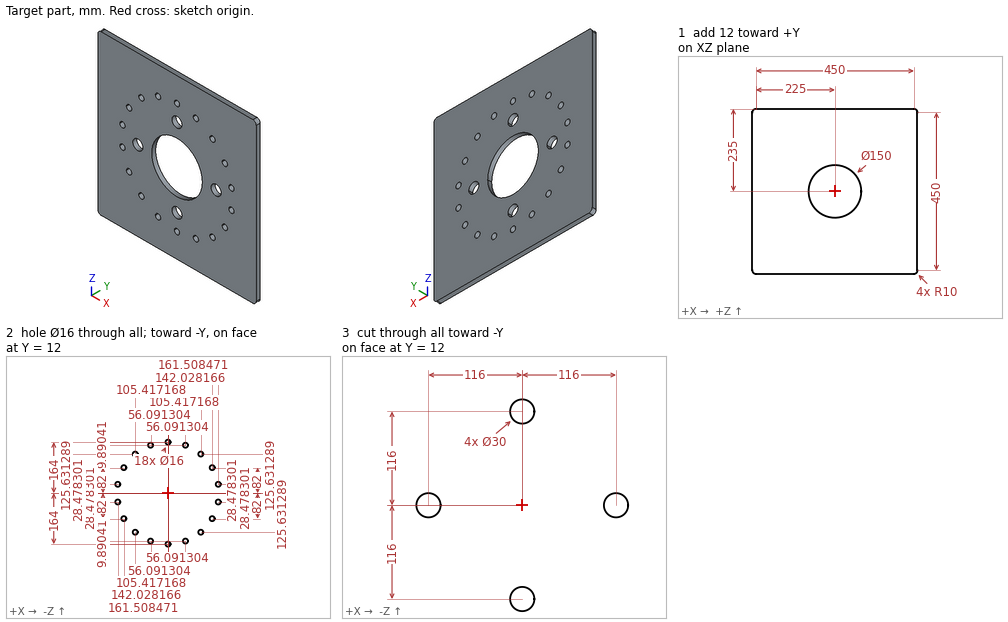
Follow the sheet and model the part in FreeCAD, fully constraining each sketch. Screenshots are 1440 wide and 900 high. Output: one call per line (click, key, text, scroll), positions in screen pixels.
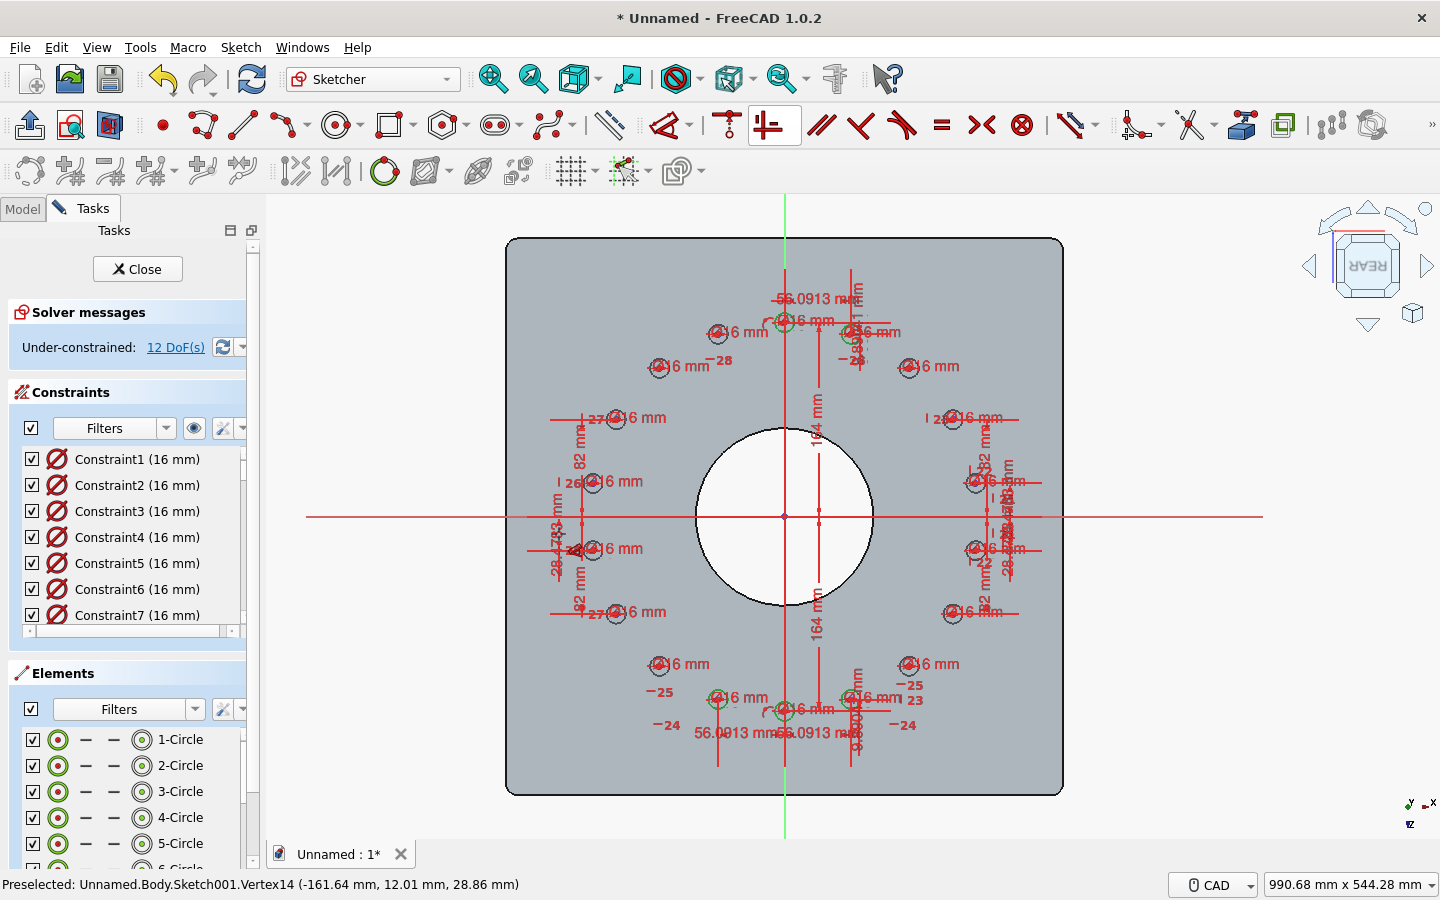
click(593, 483)
click(559, 500)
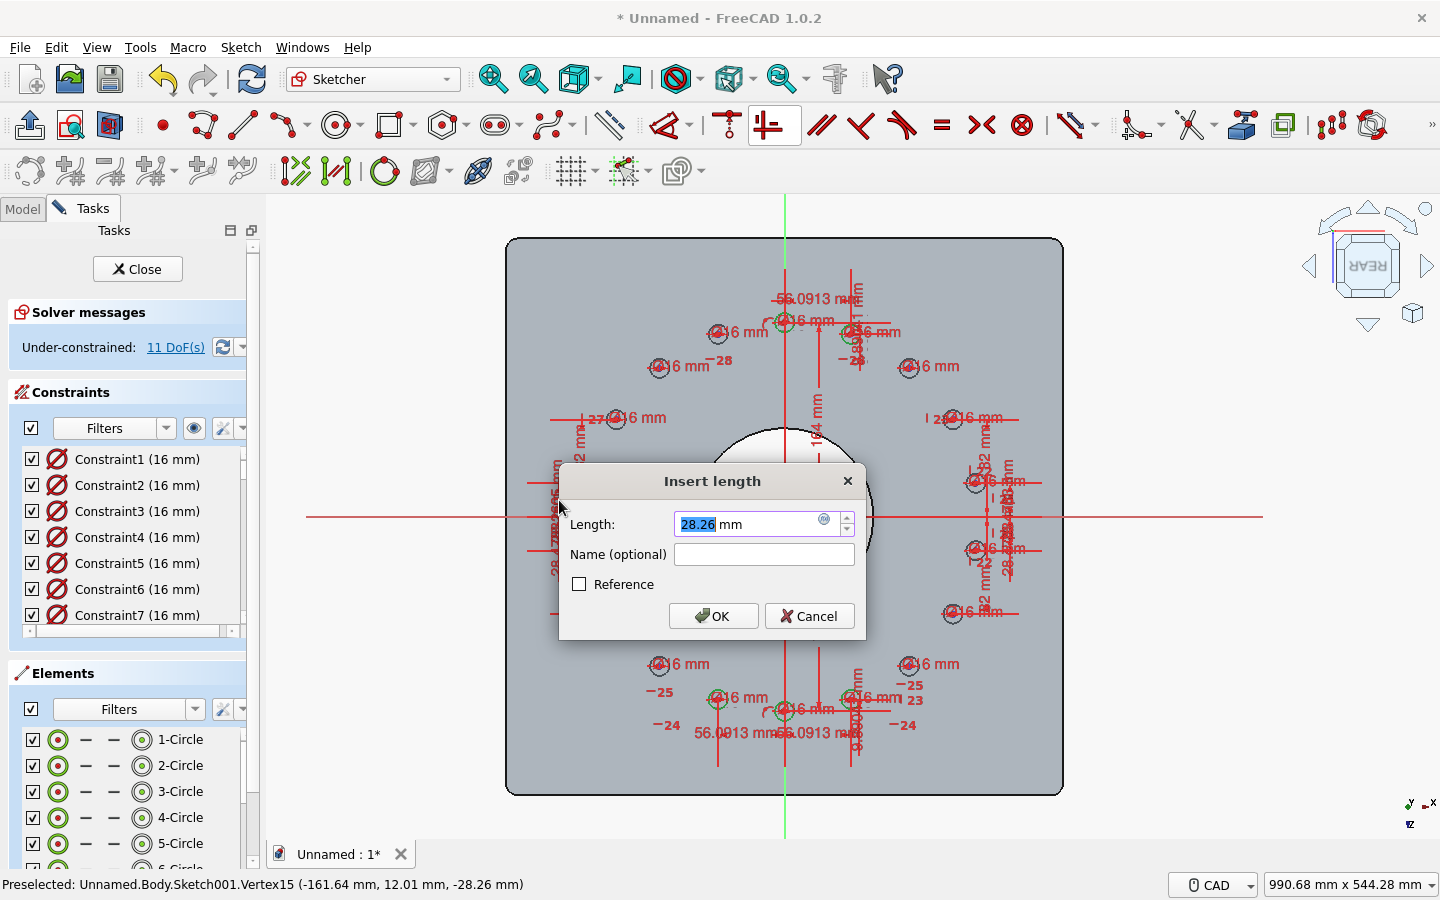
text(28.478301)
key(Return)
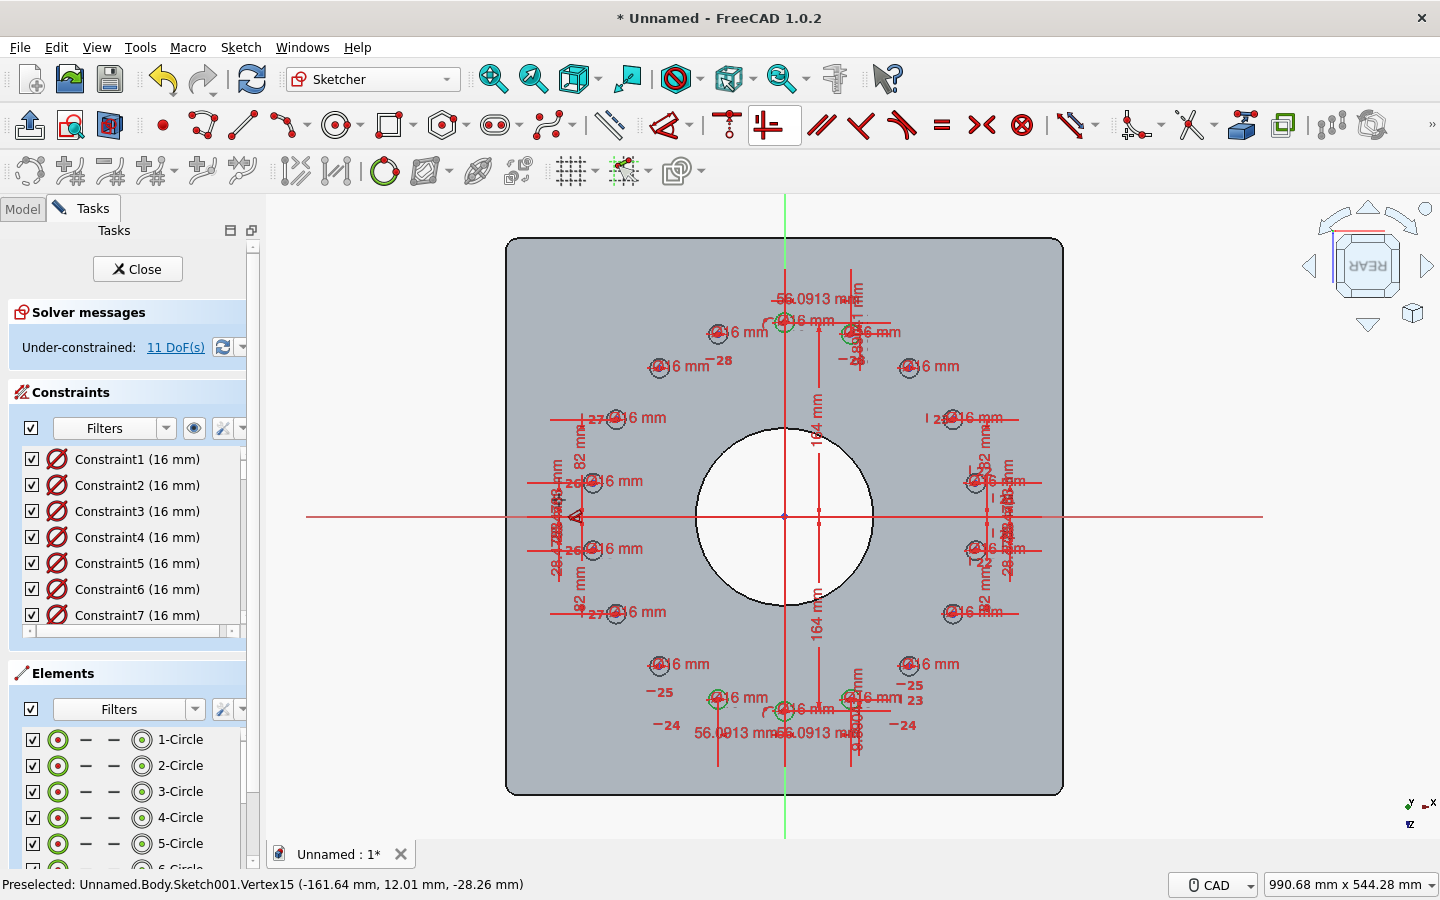
click(718, 334)
click(736, 300)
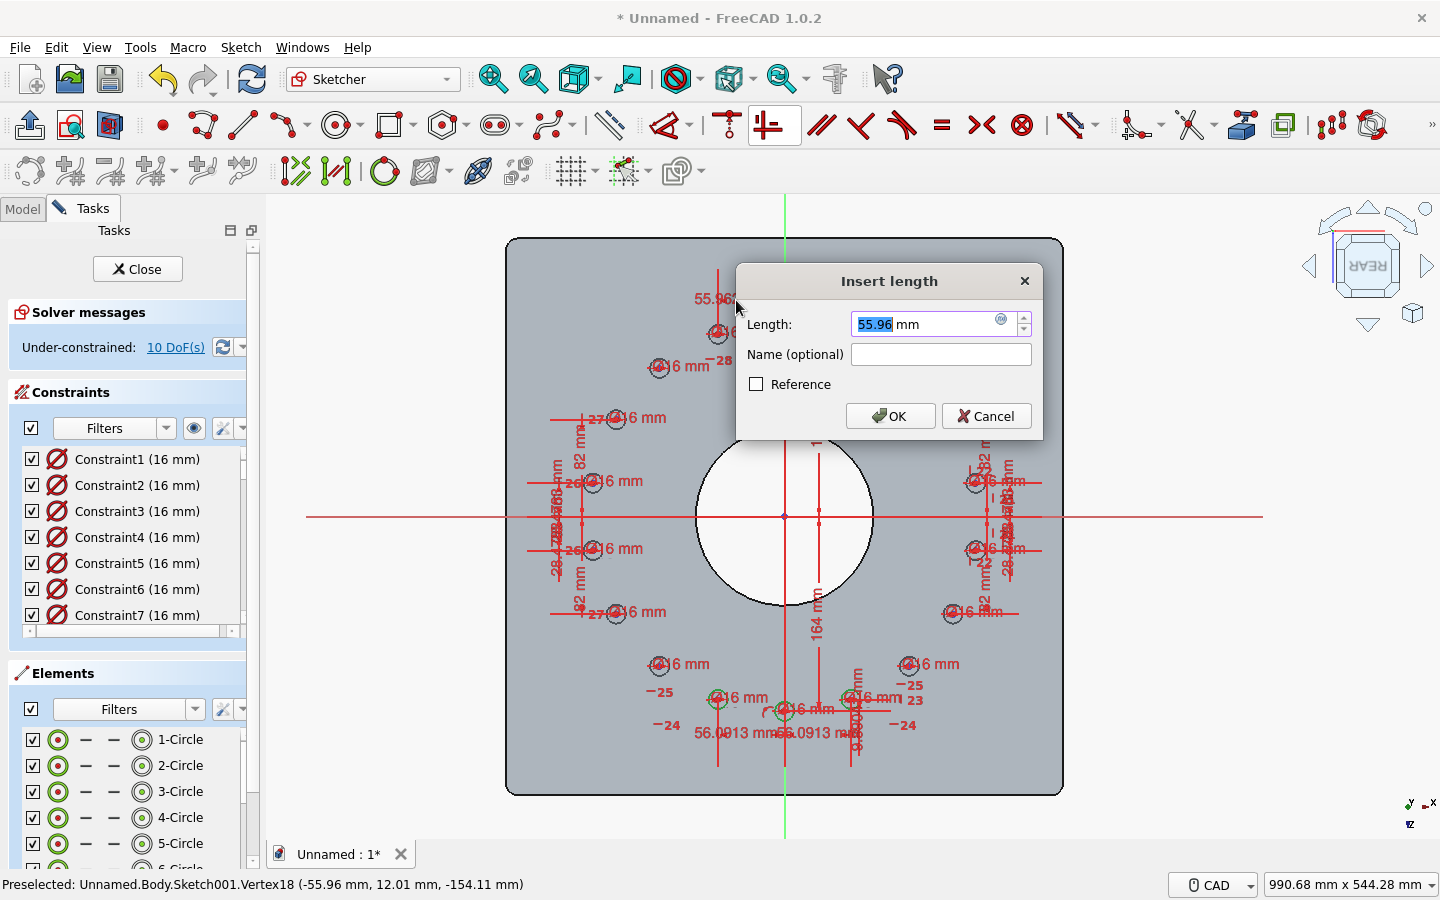
text(56.091304)
key(Return)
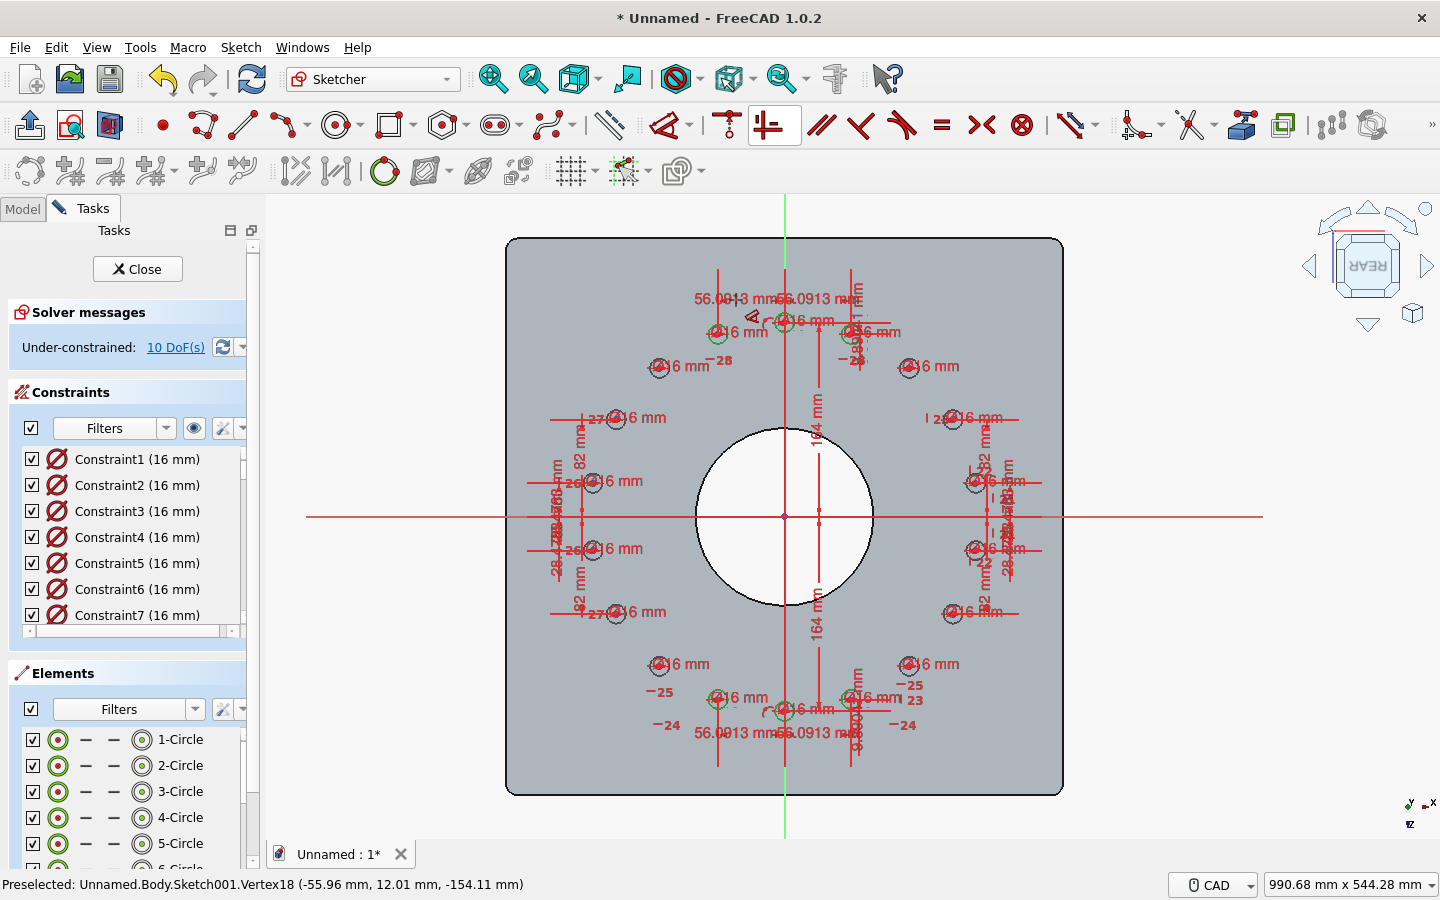
click(909, 368)
click(847, 551)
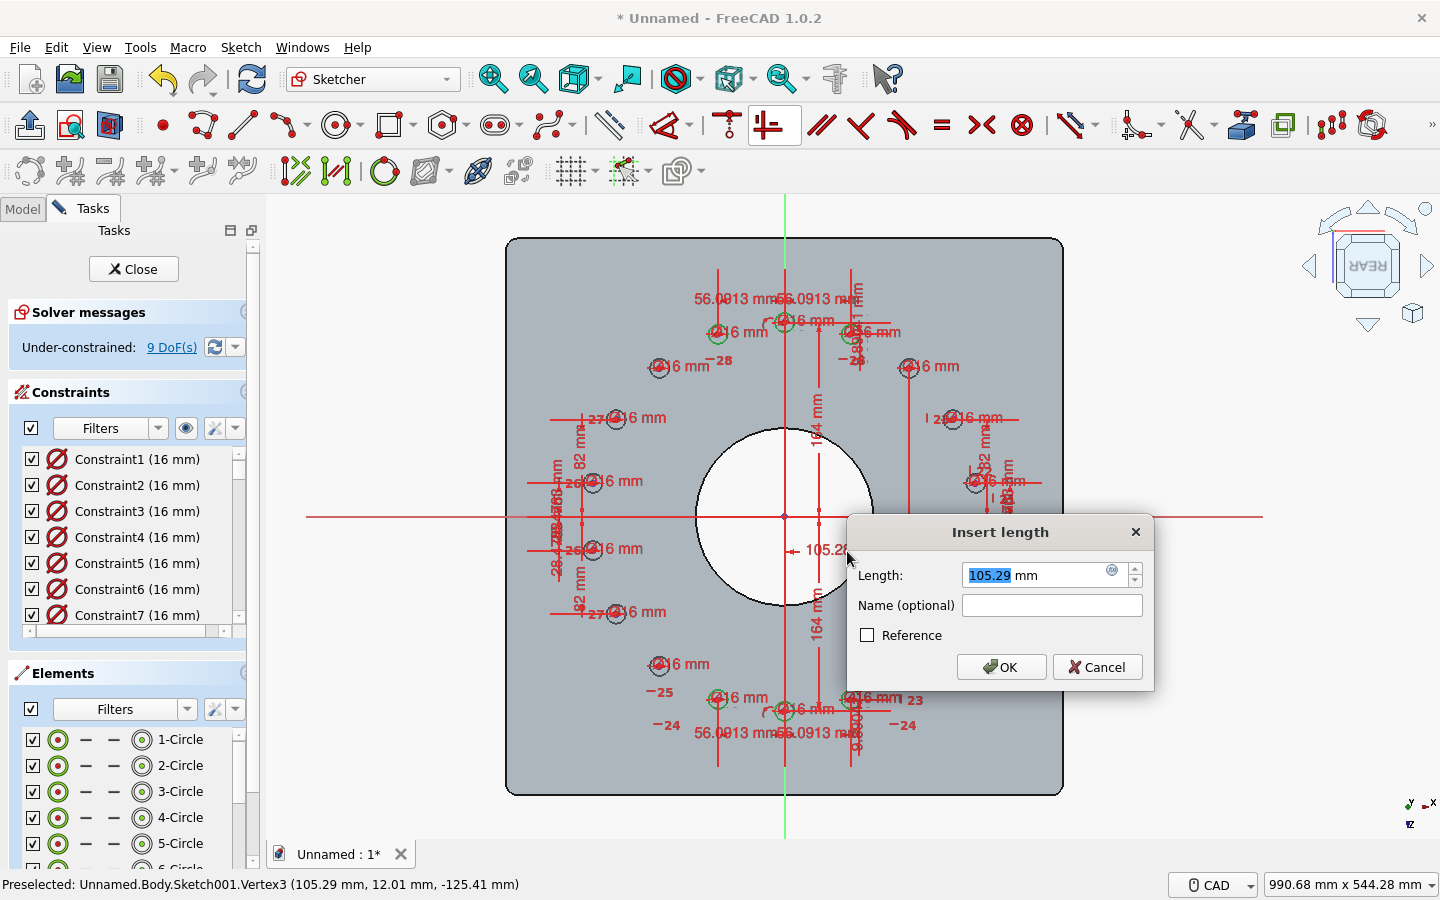
text(105.417168)
key(Return)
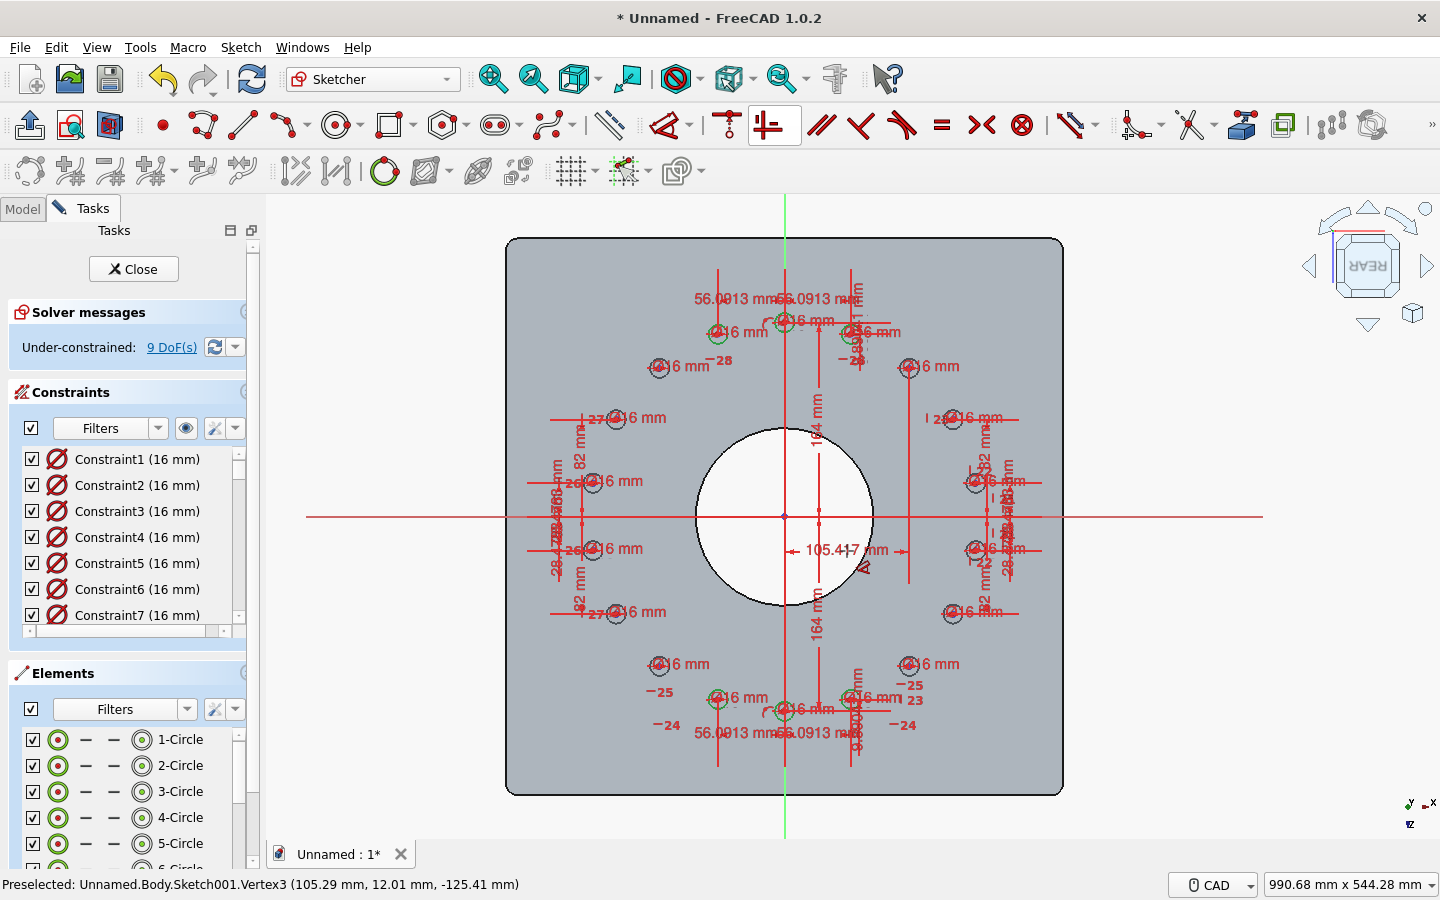
click(909, 368)
click(943, 477)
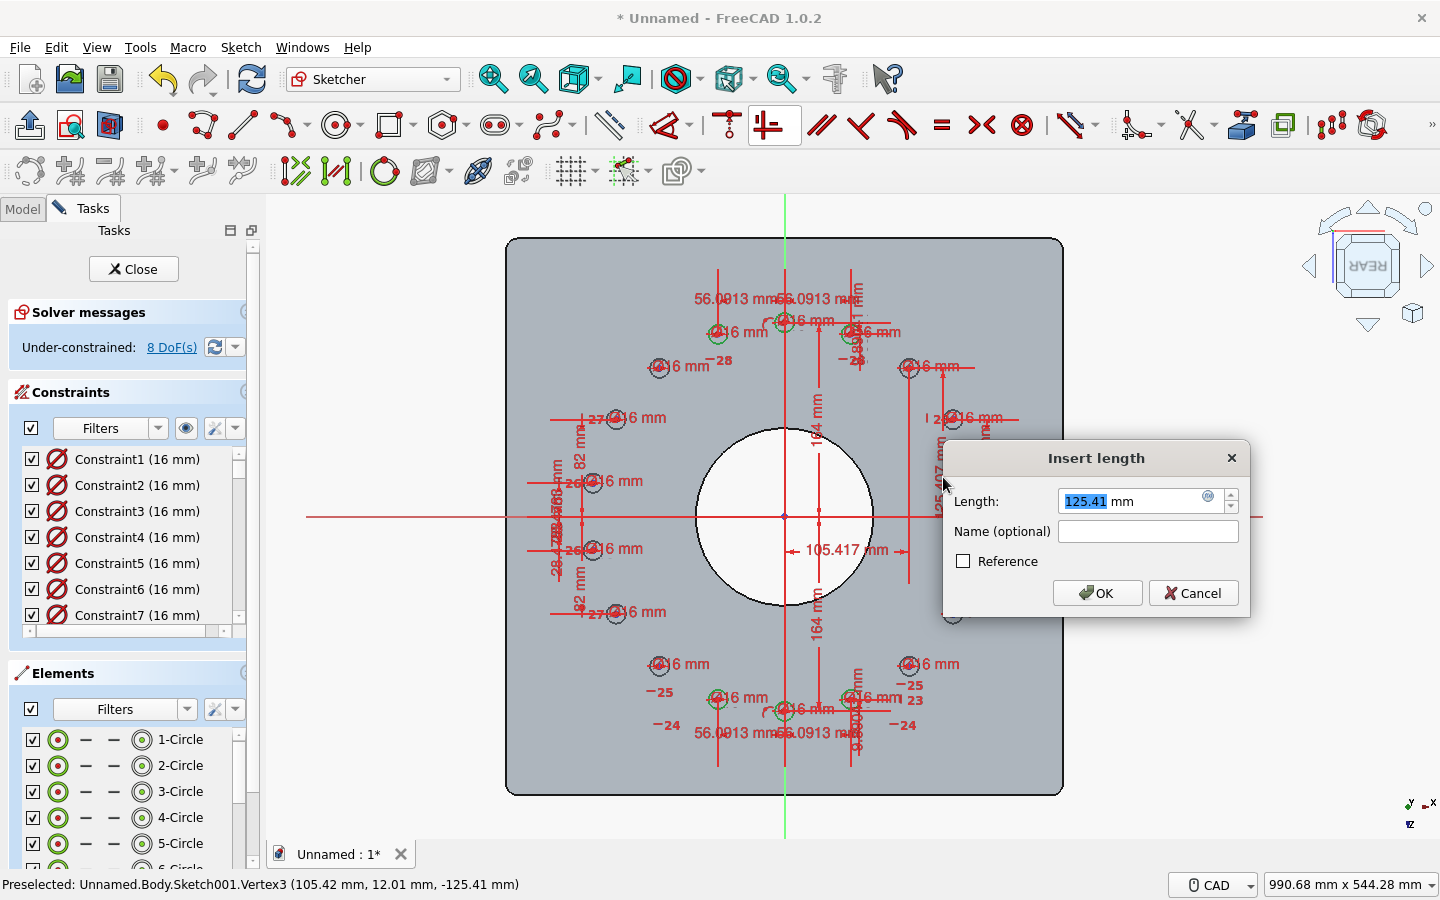
text(125.631289)
key(Return)